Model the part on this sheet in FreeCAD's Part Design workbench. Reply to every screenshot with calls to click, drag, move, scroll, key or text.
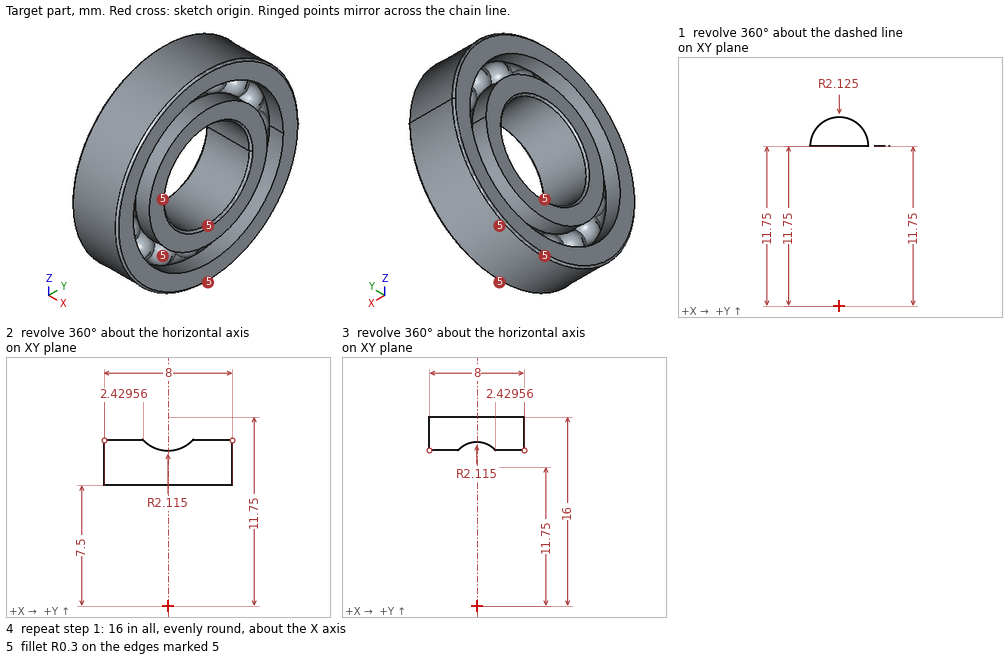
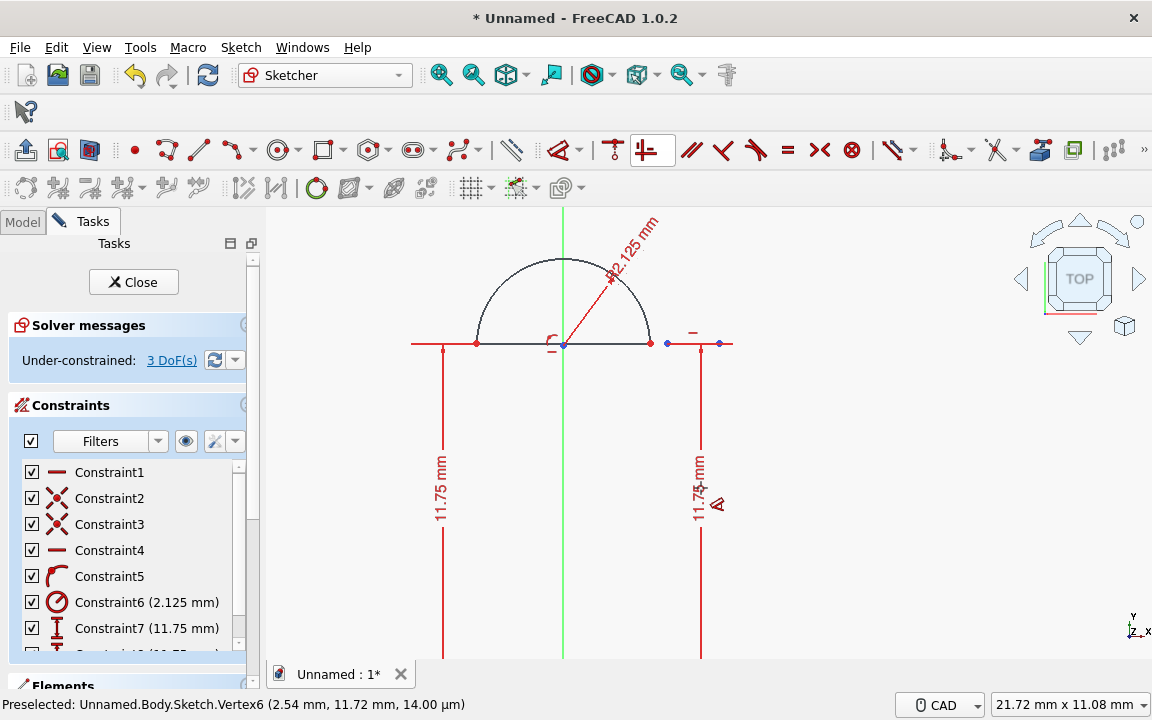
click(563, 346)
click(529, 488)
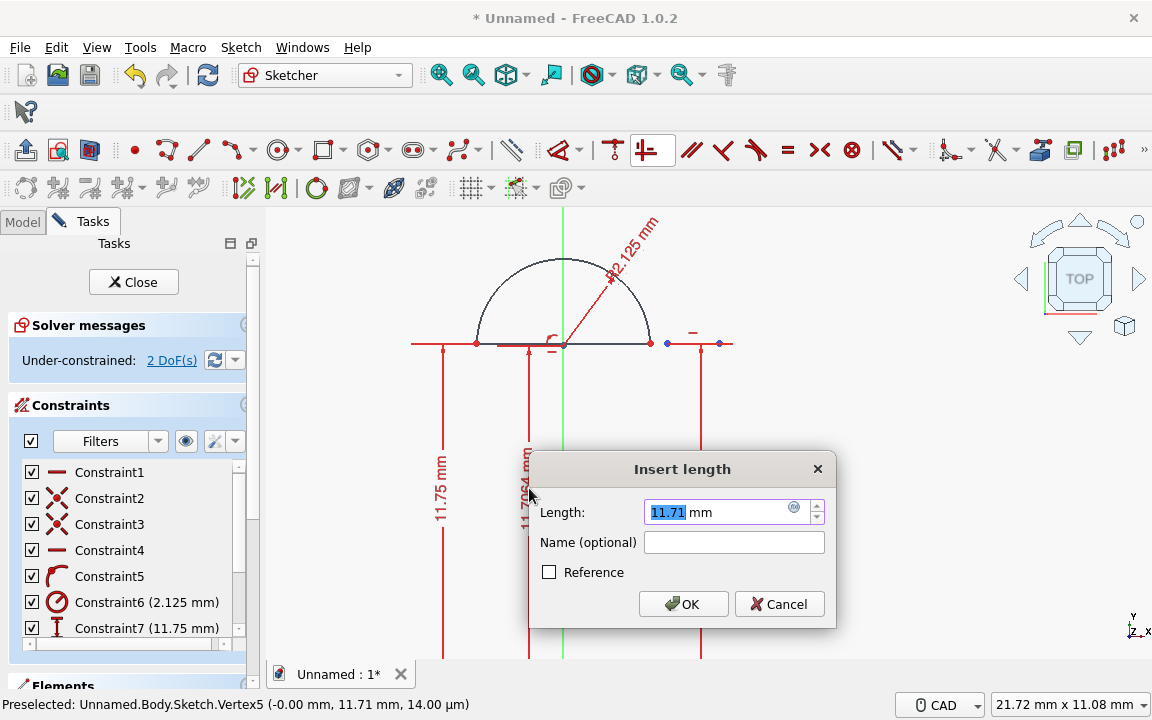
text(11.75)
key(Return)
key(Escape)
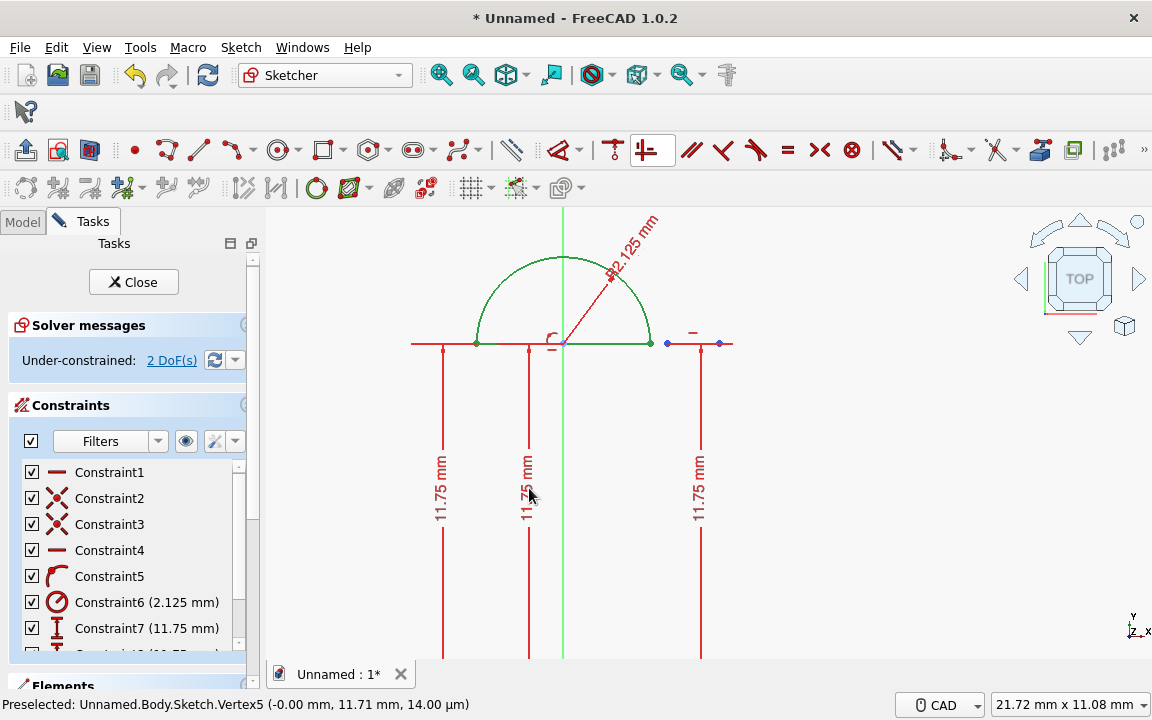
click(134, 282)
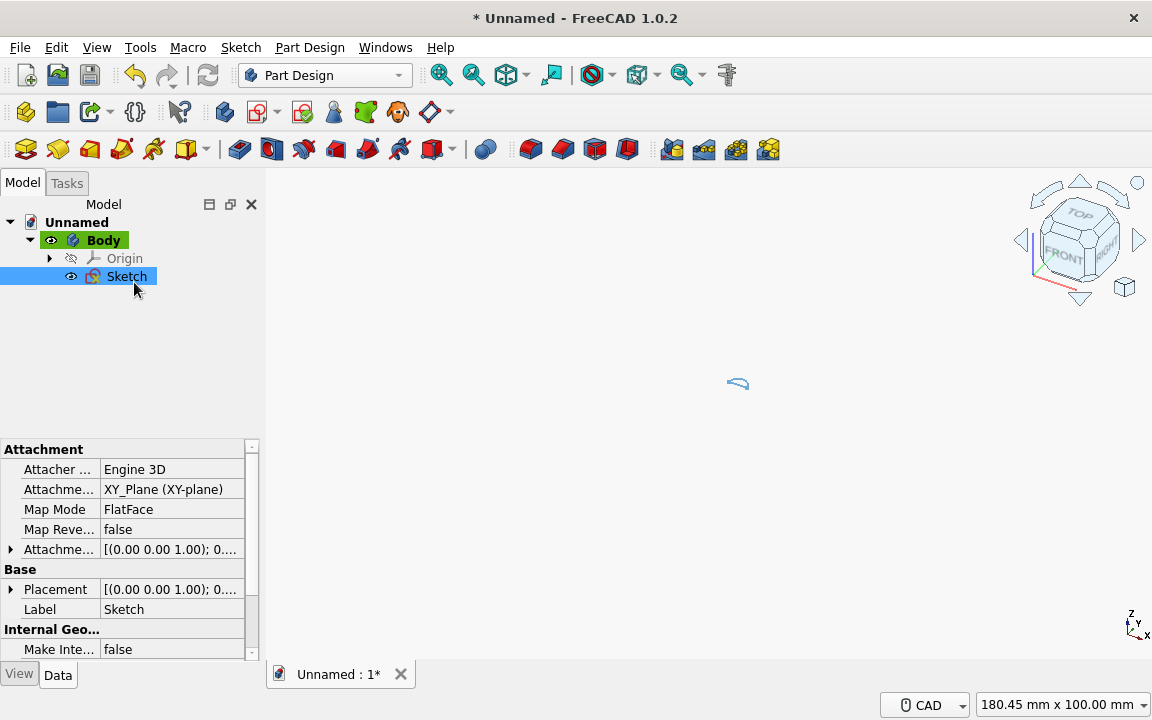
click(58, 150)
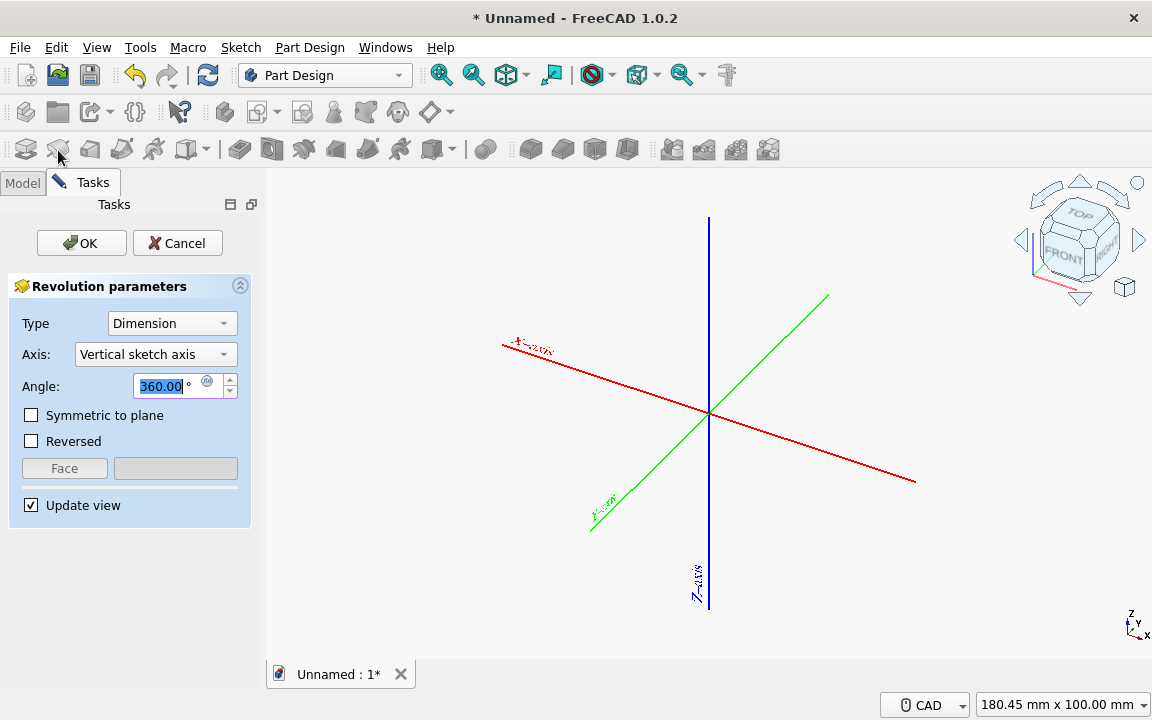
click(156, 354)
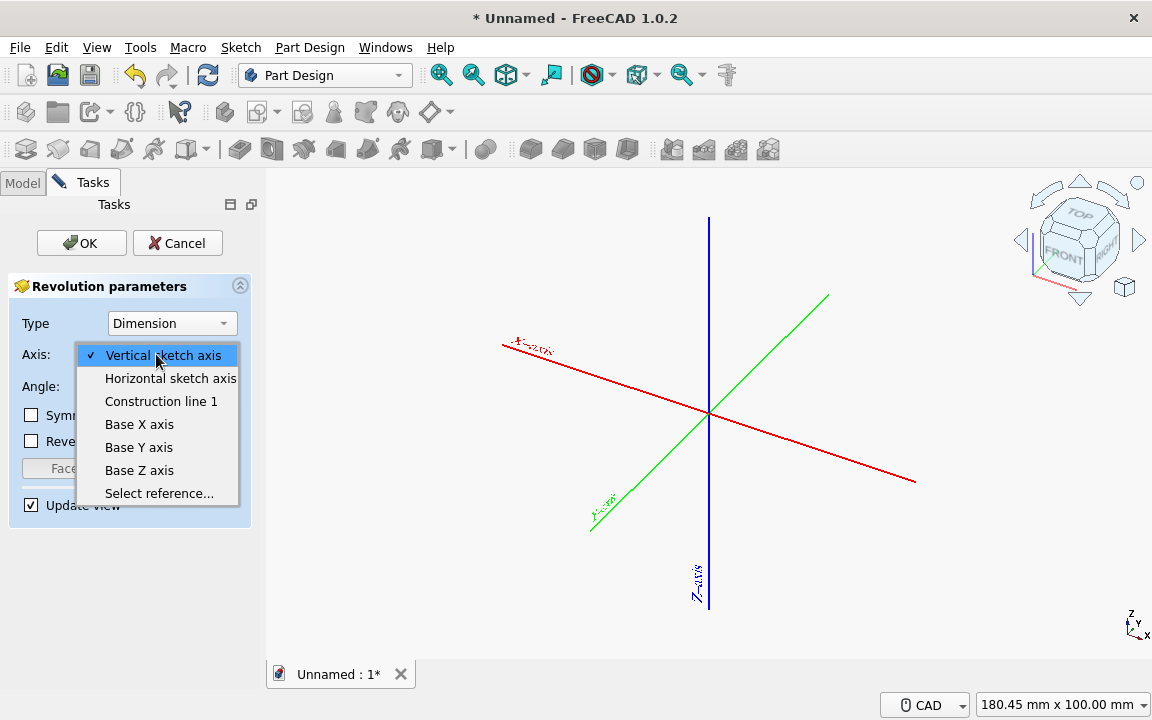
click(156, 402)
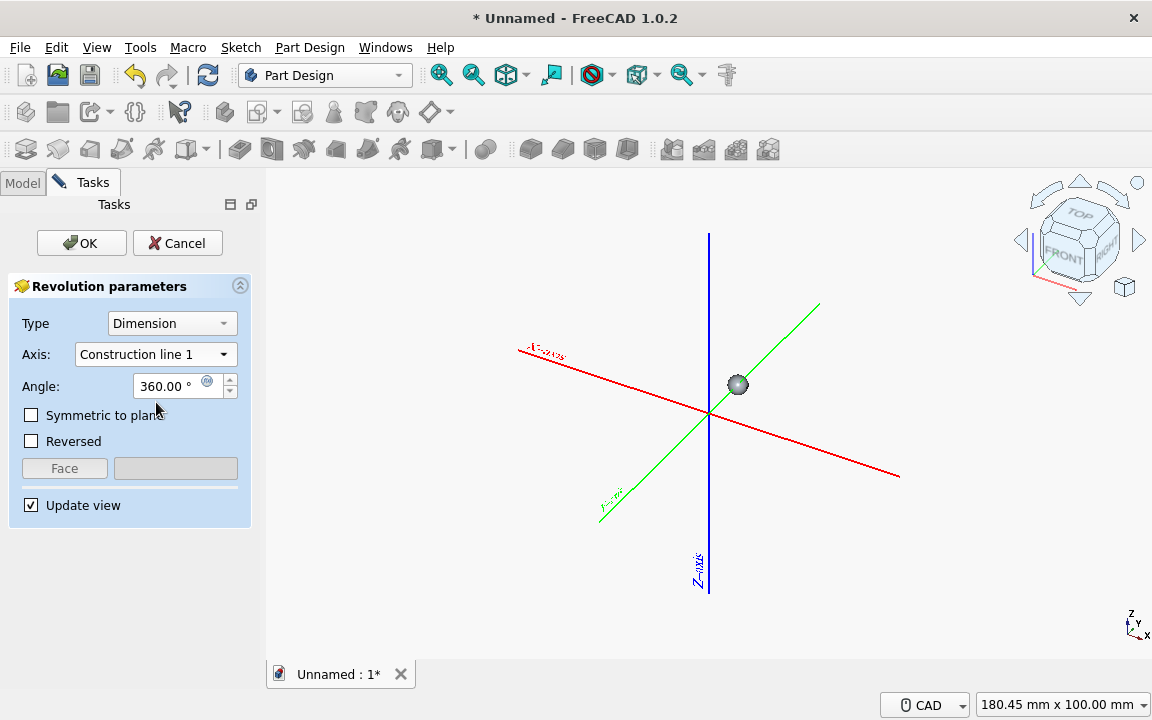
click(82, 243)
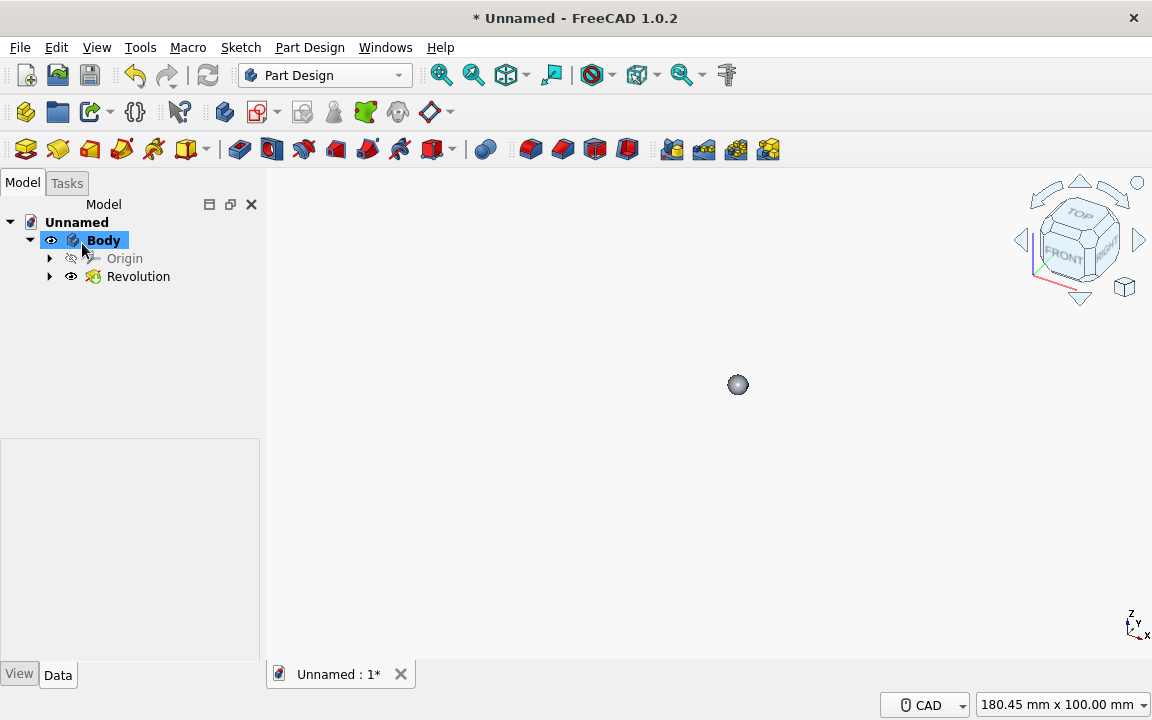
click(442, 76)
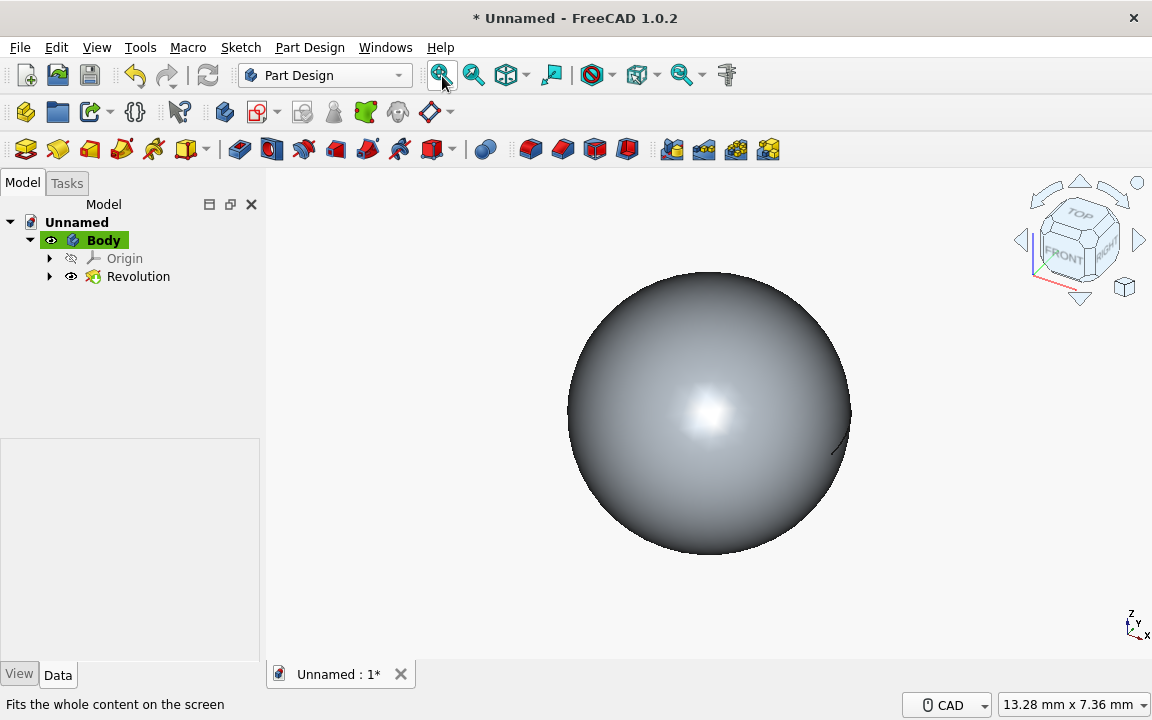
click(258, 112)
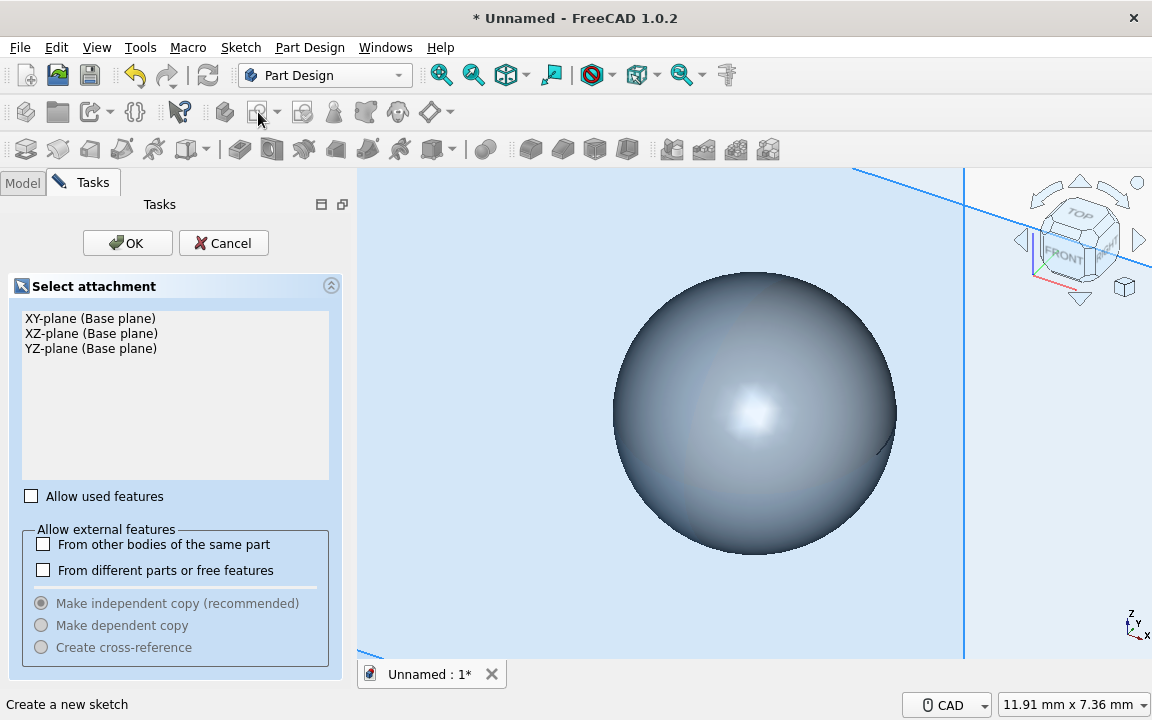
click(82, 318)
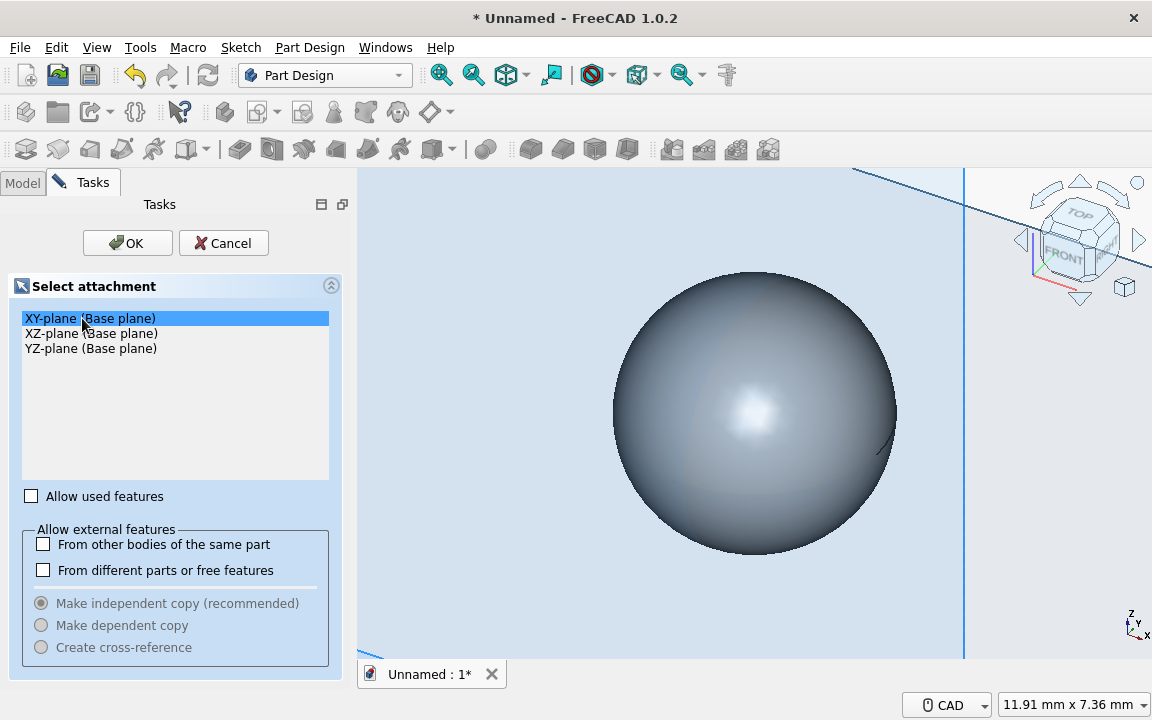
click(128, 243)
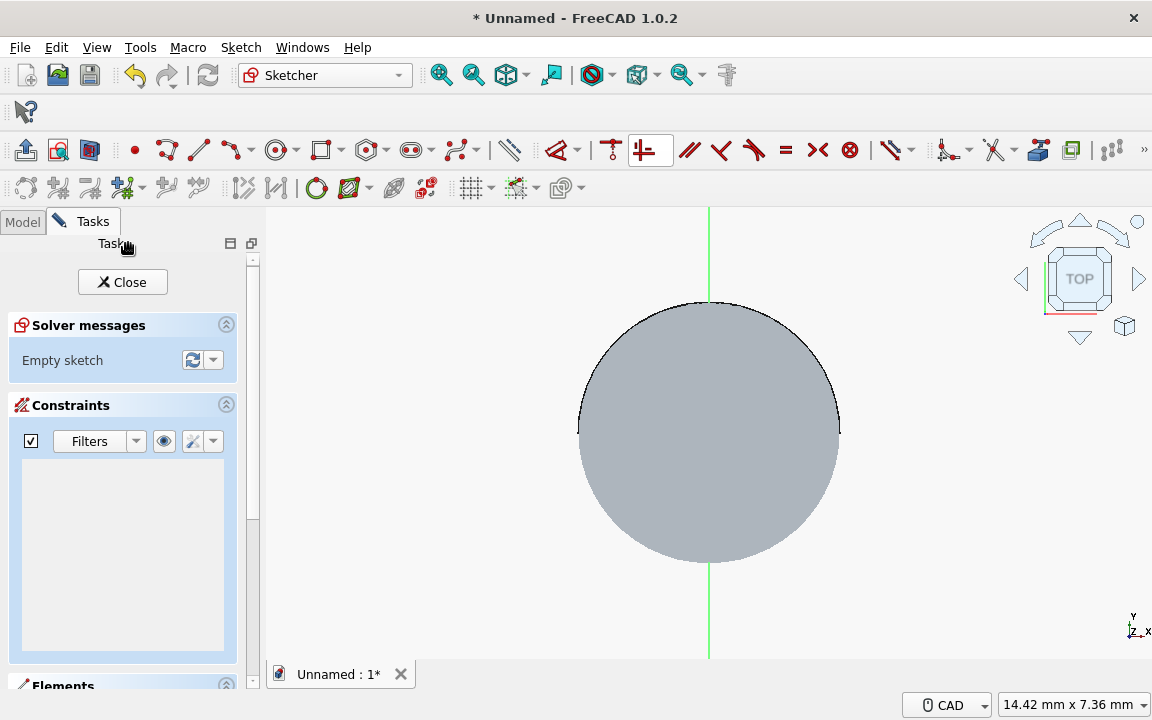
click(90, 150)